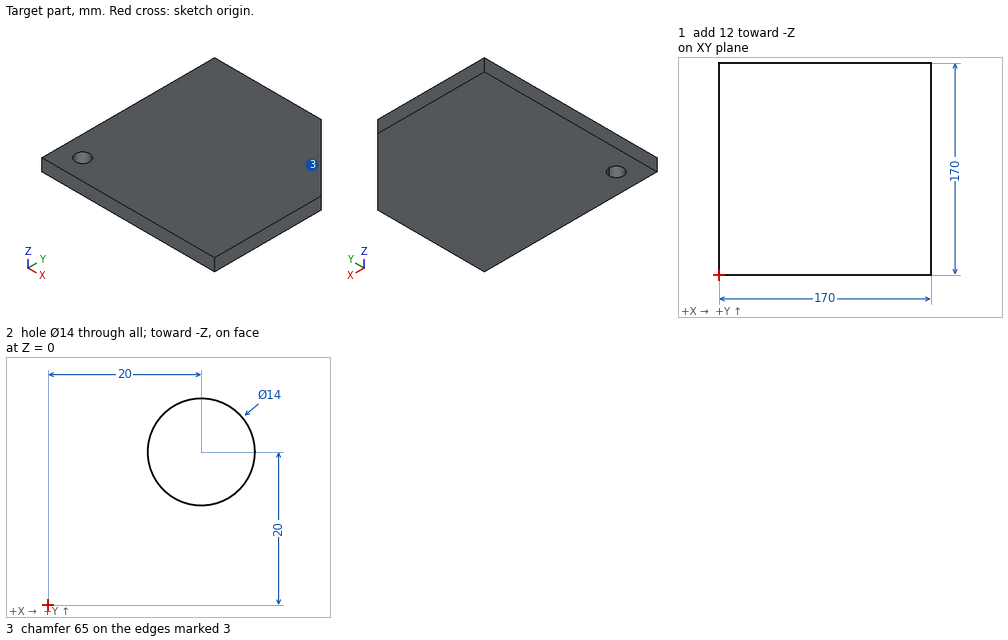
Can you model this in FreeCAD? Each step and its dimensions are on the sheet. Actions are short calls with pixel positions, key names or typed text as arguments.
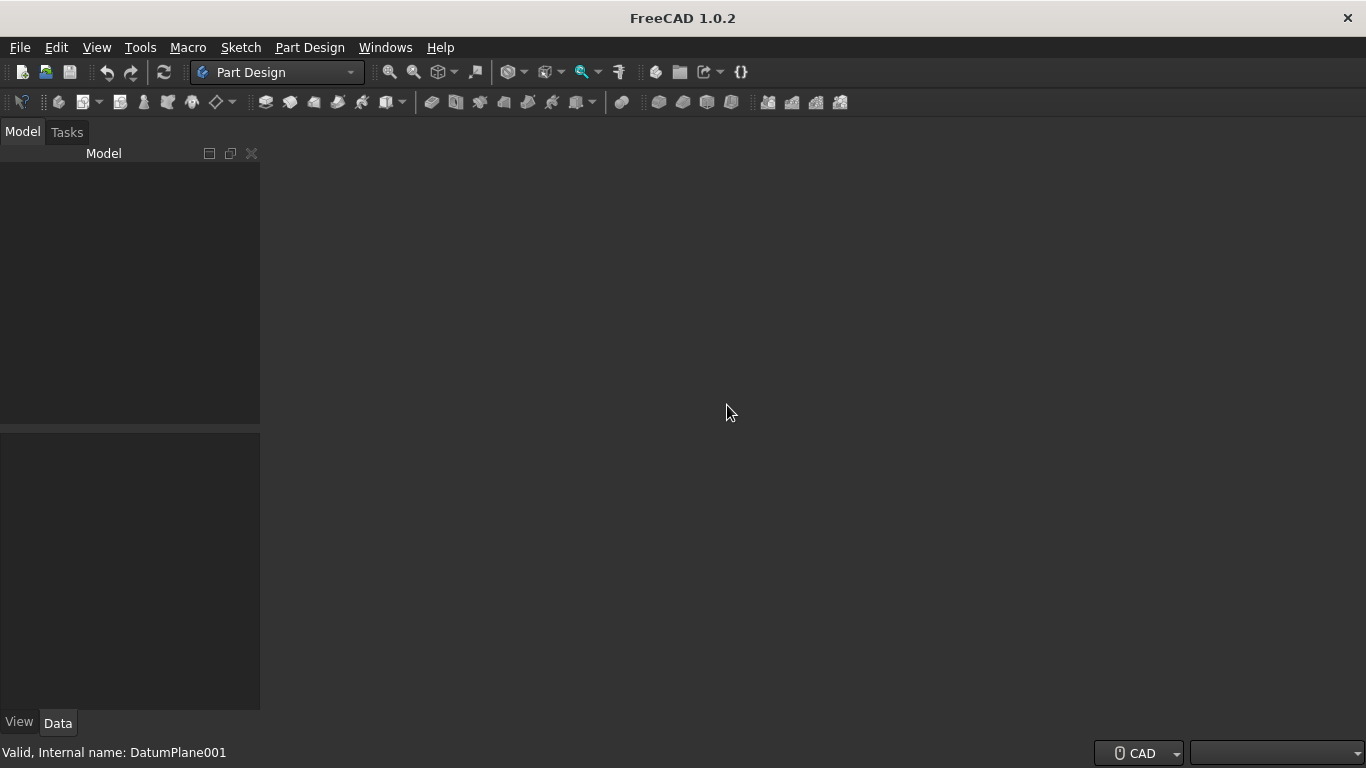
click(22, 72)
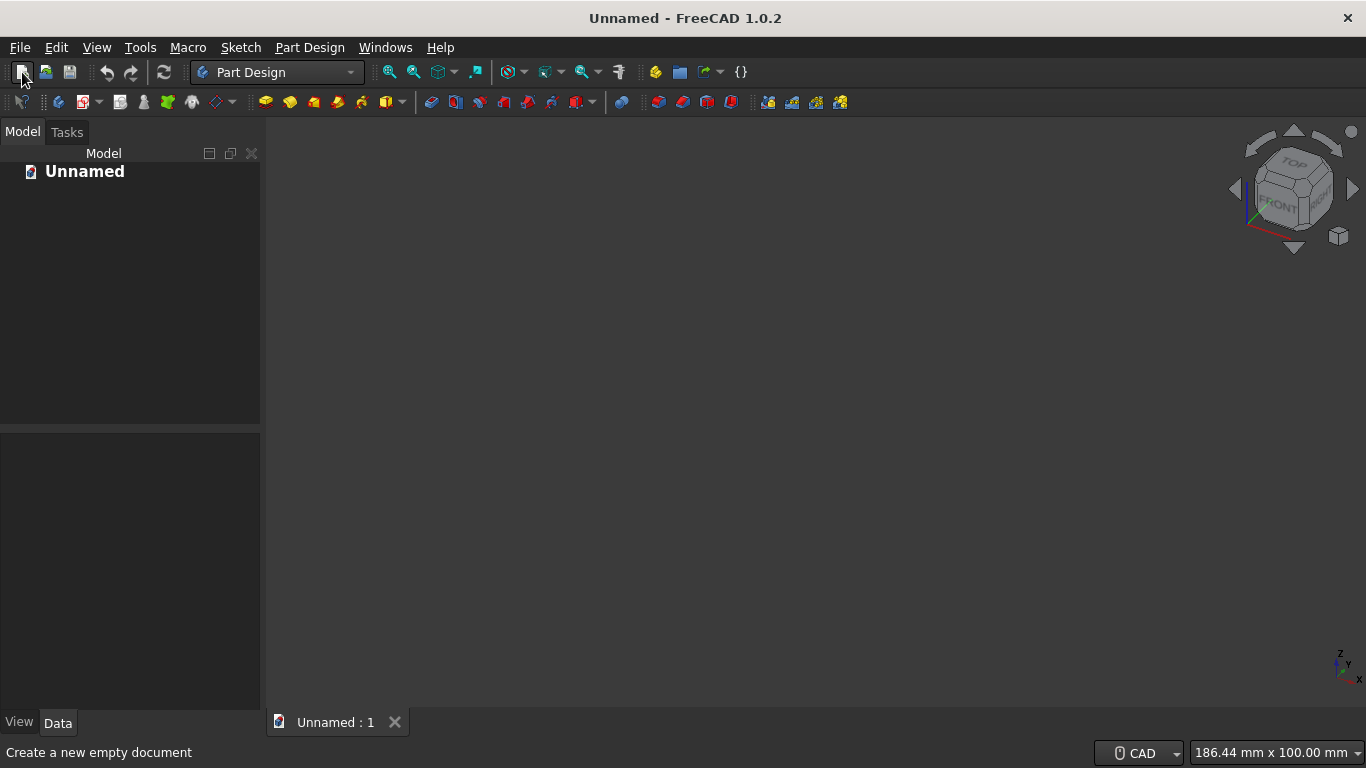
click(84, 102)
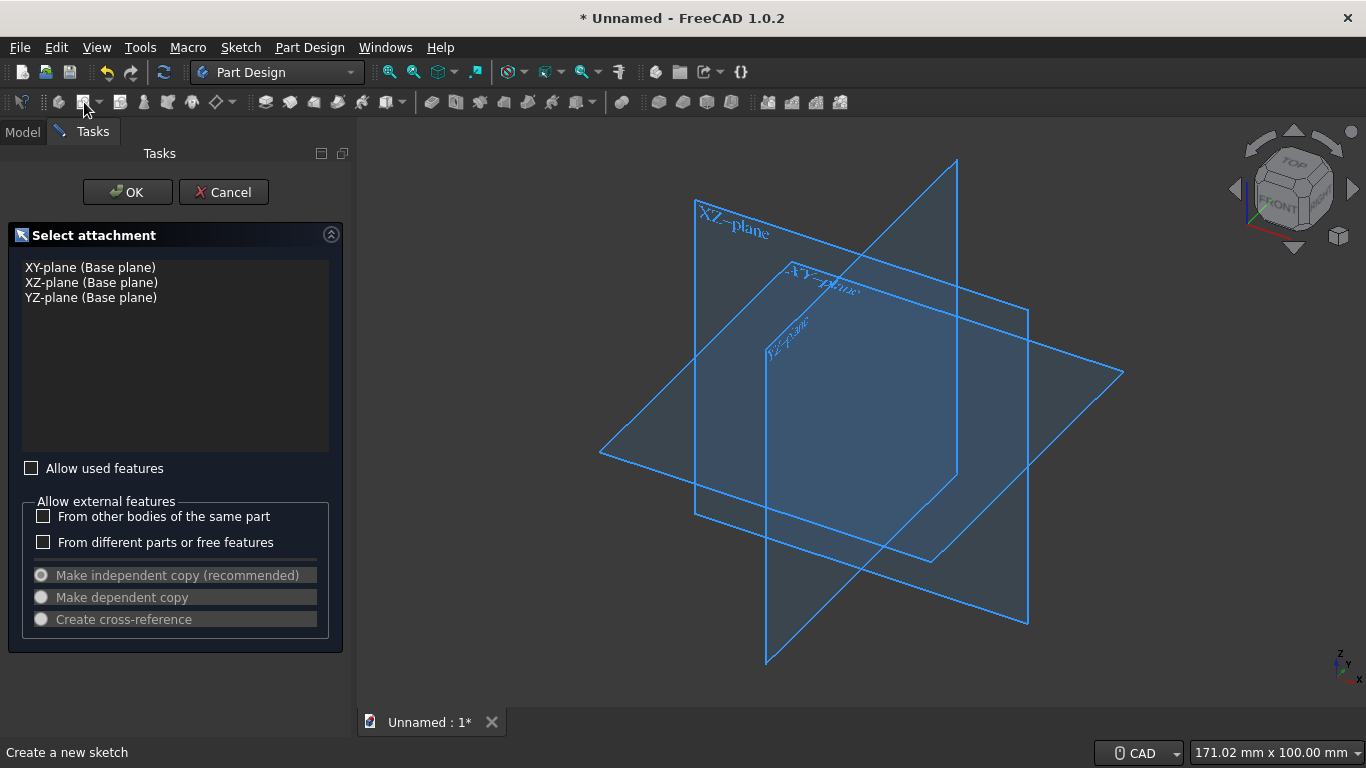
click(82, 268)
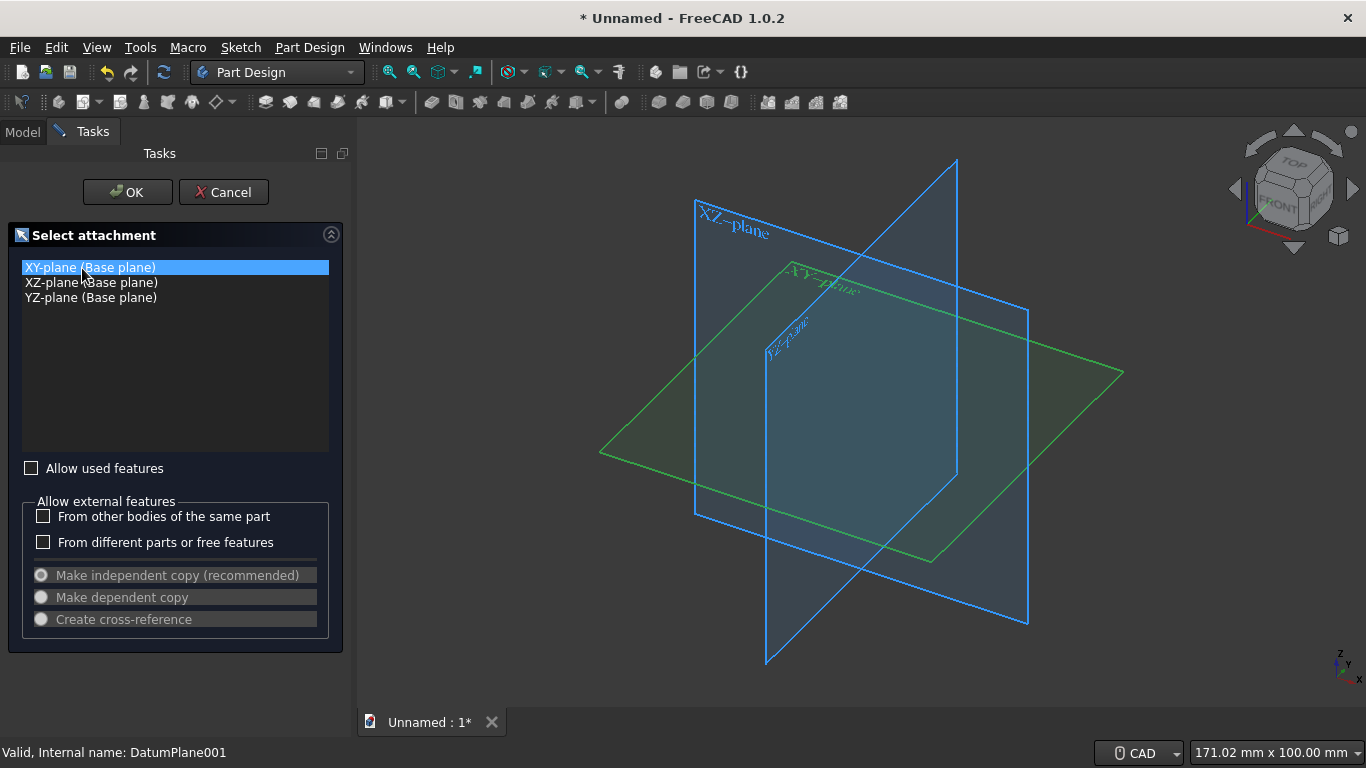
click(128, 192)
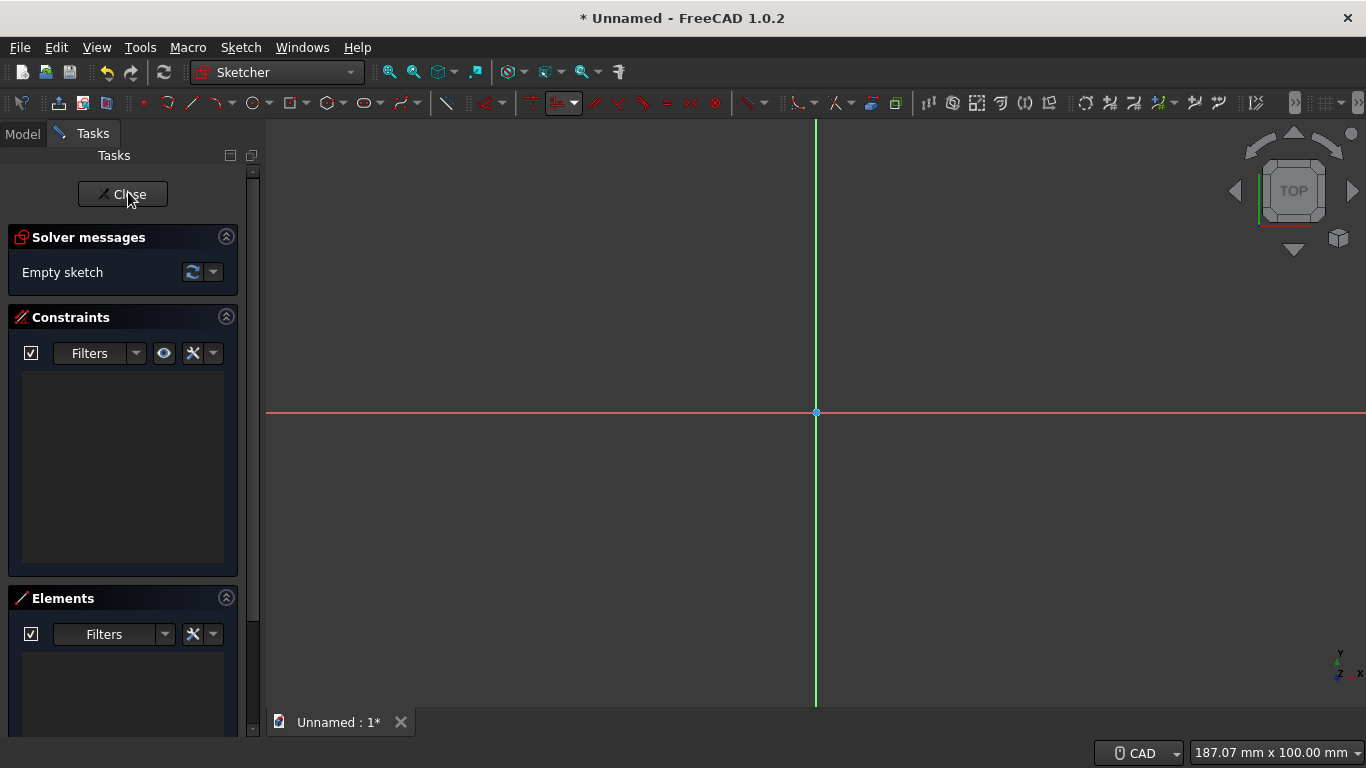
scroll(417, 679, down, 5)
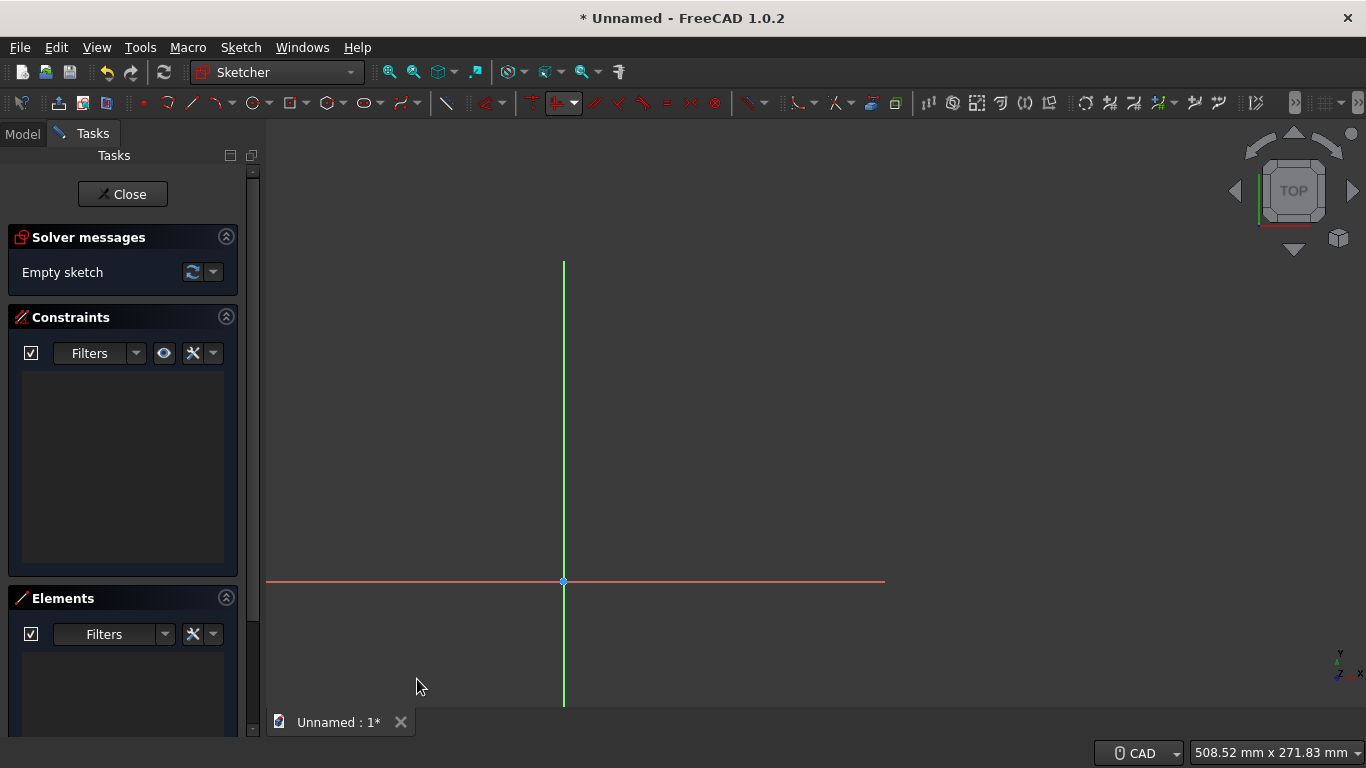
key(g)
key(r)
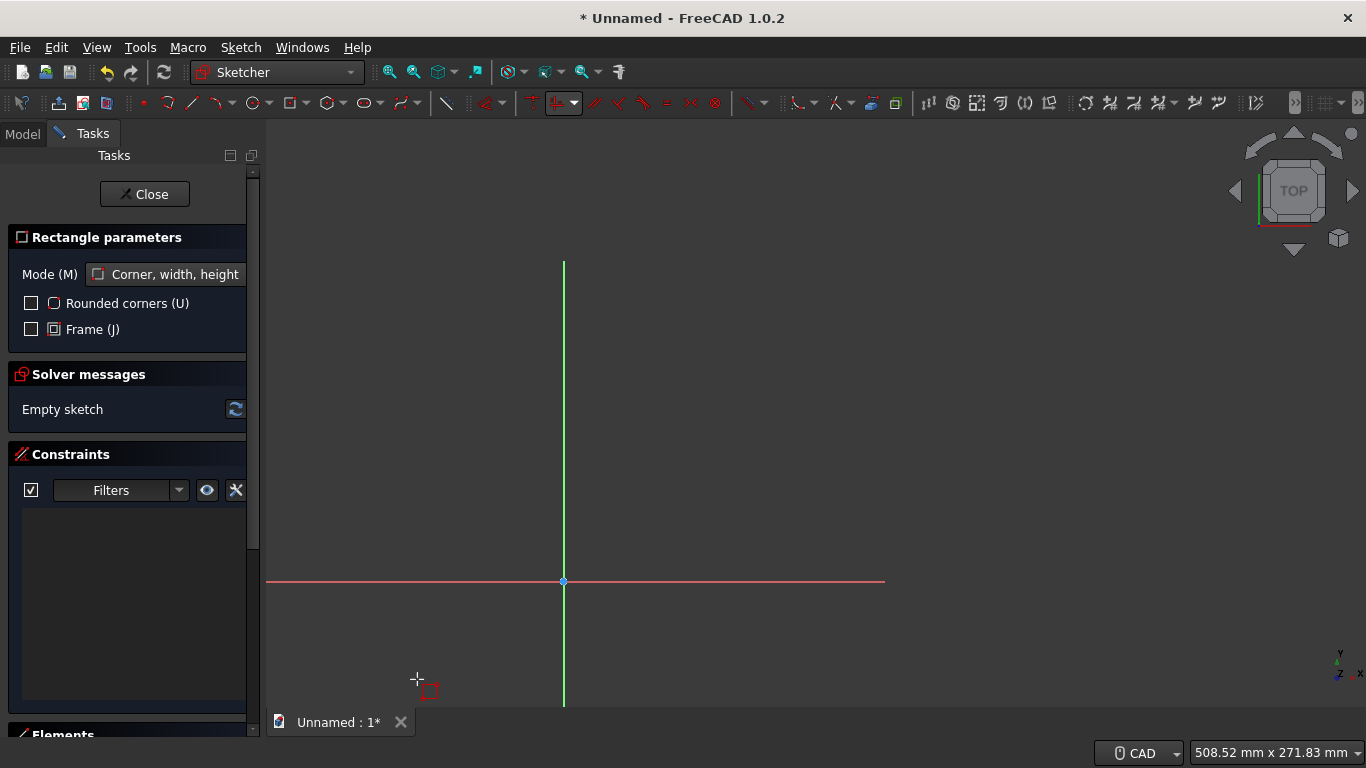
click(564, 582)
click(932, 214)
key(Escape)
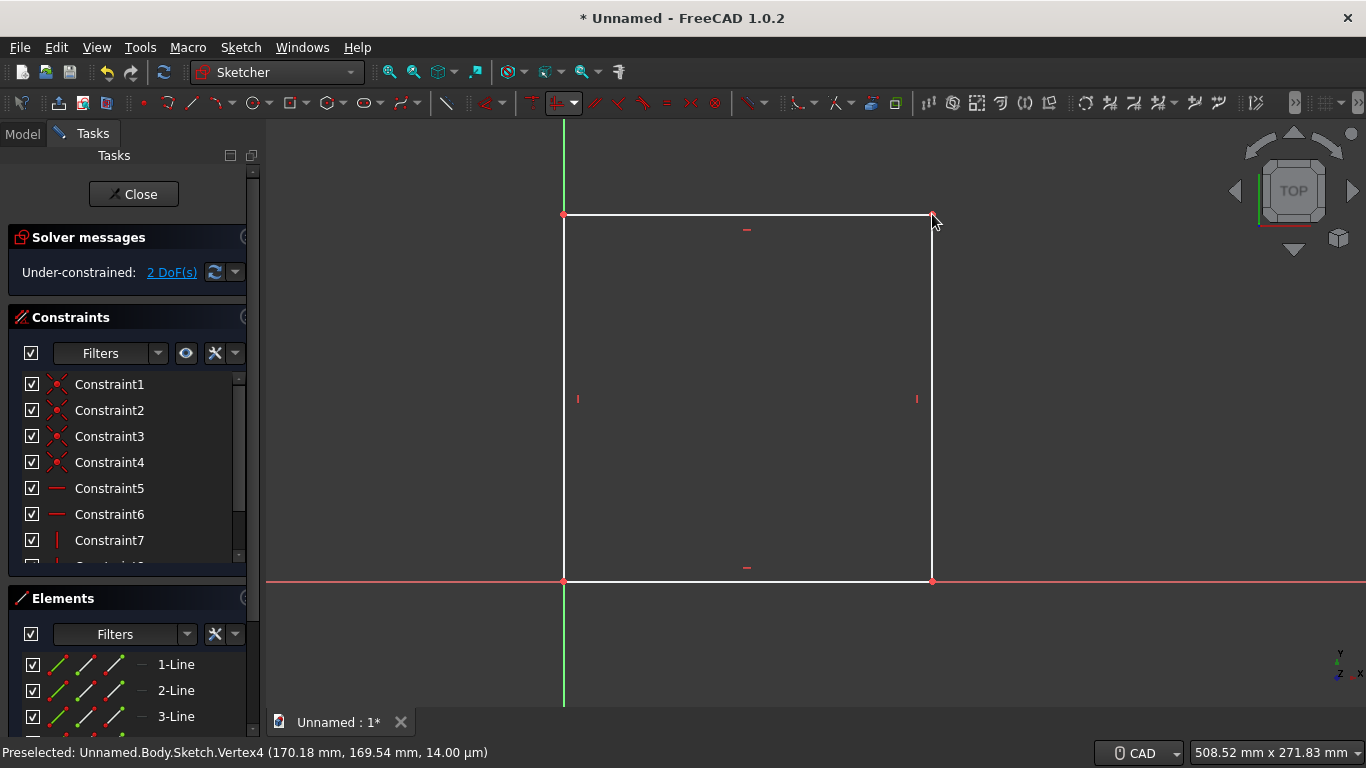
click(674, 582)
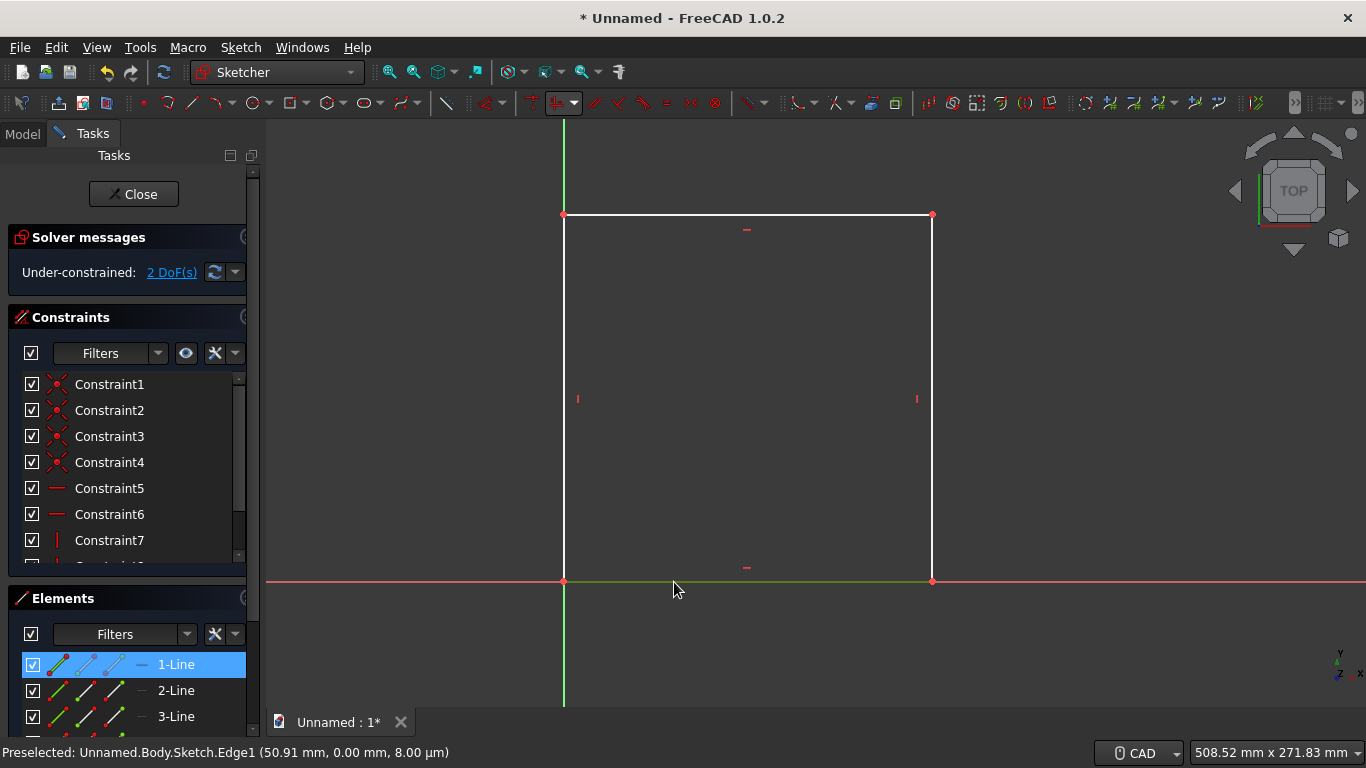
key(l)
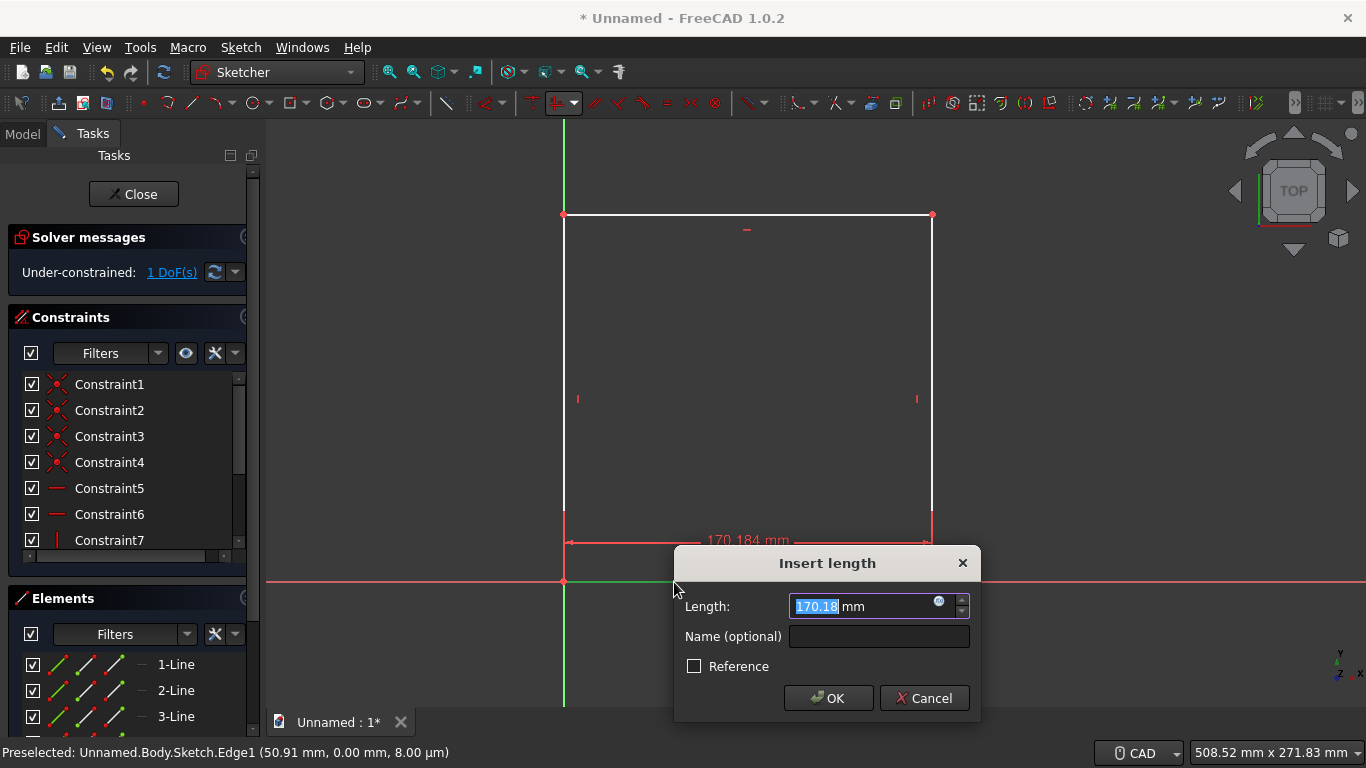
text(170)
key(Return)